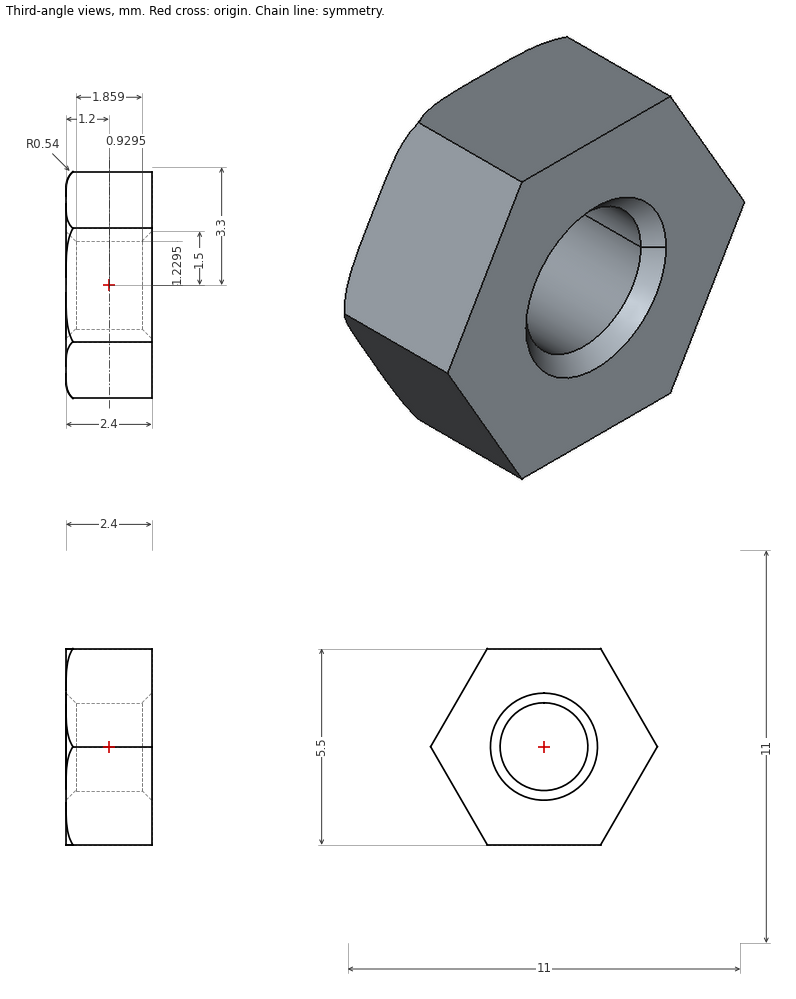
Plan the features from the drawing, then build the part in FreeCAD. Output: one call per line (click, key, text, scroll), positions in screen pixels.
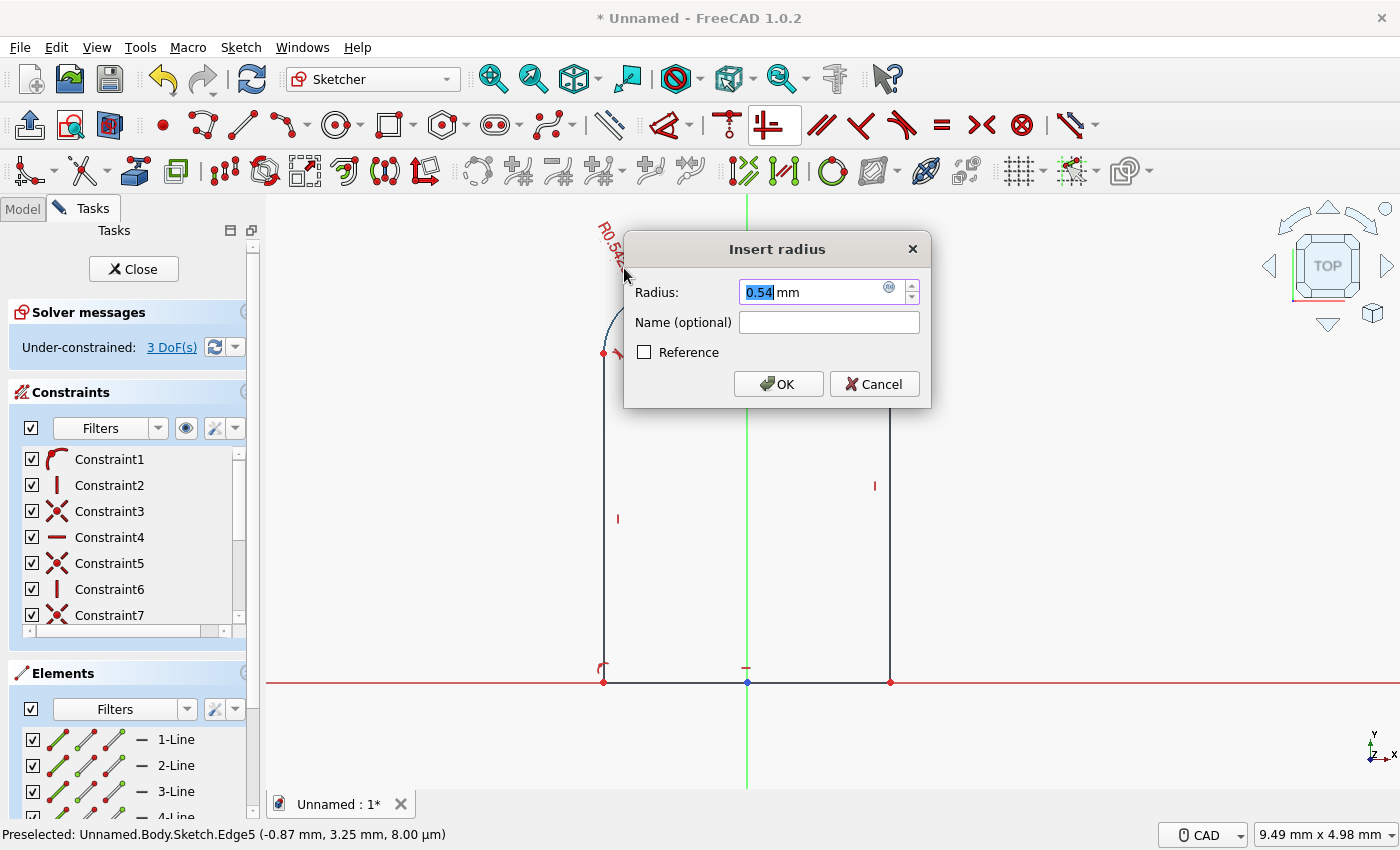
text(0.54)
key(Return)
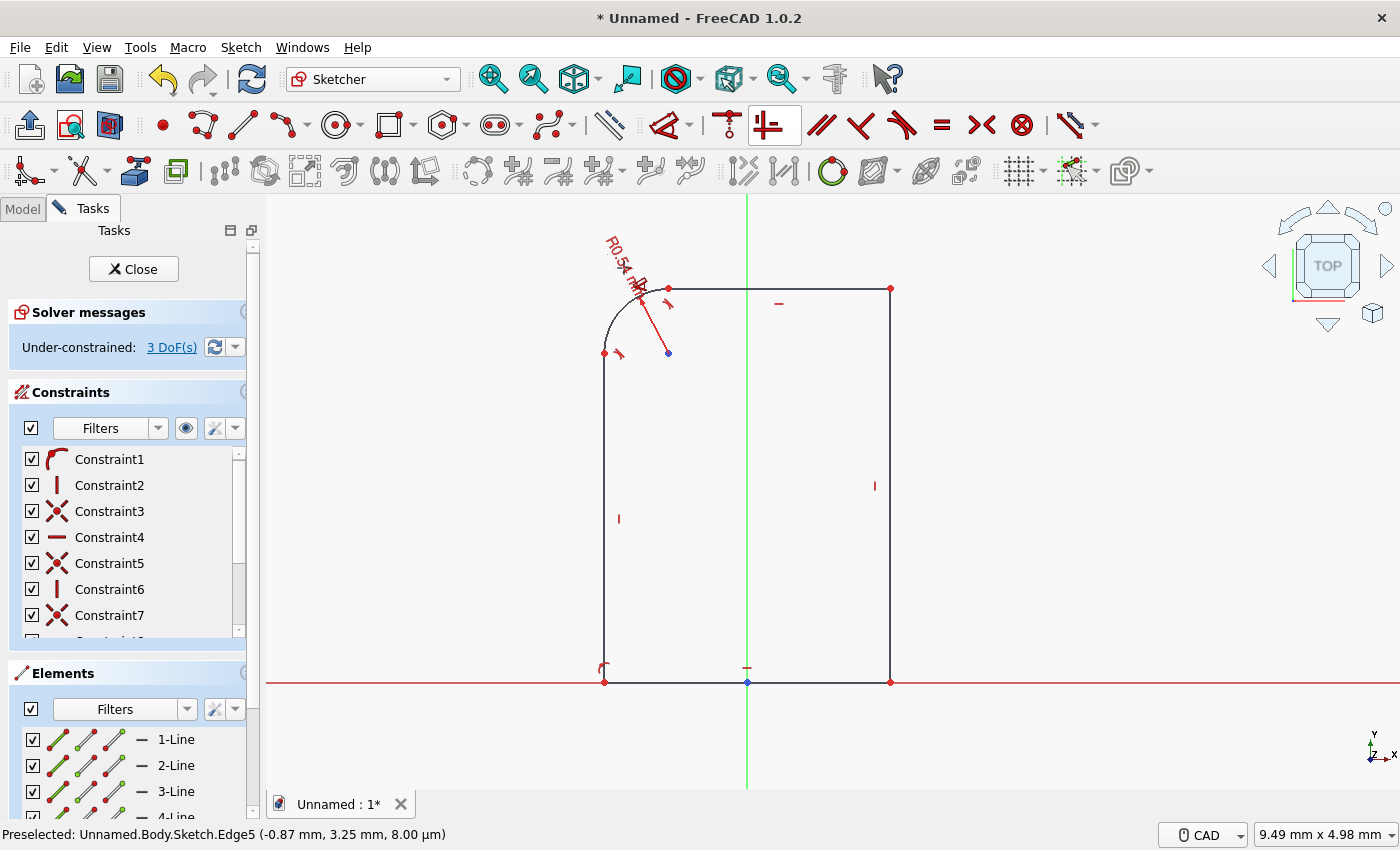
click(690, 683)
click(681, 717)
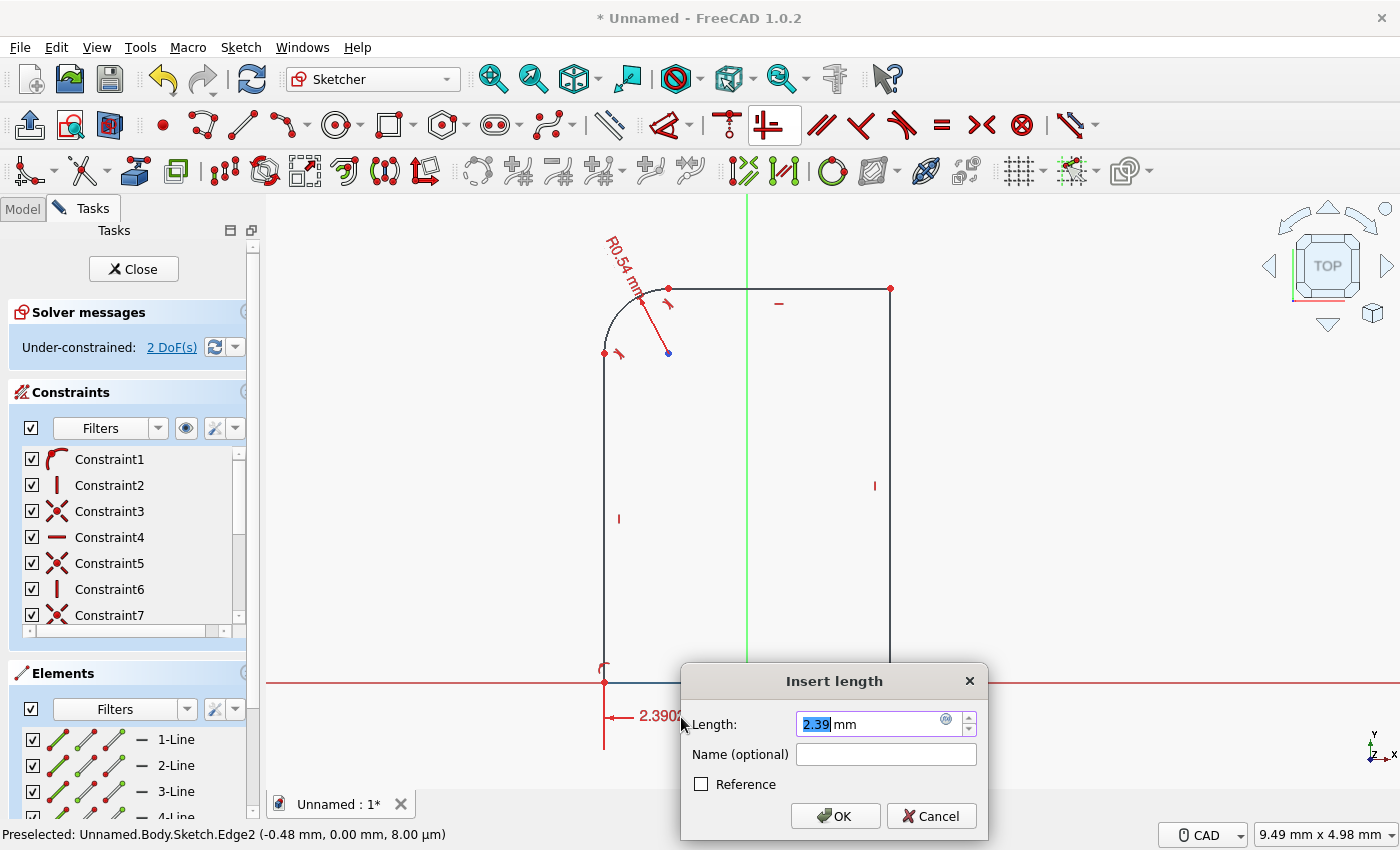
text(2.4)
key(Return)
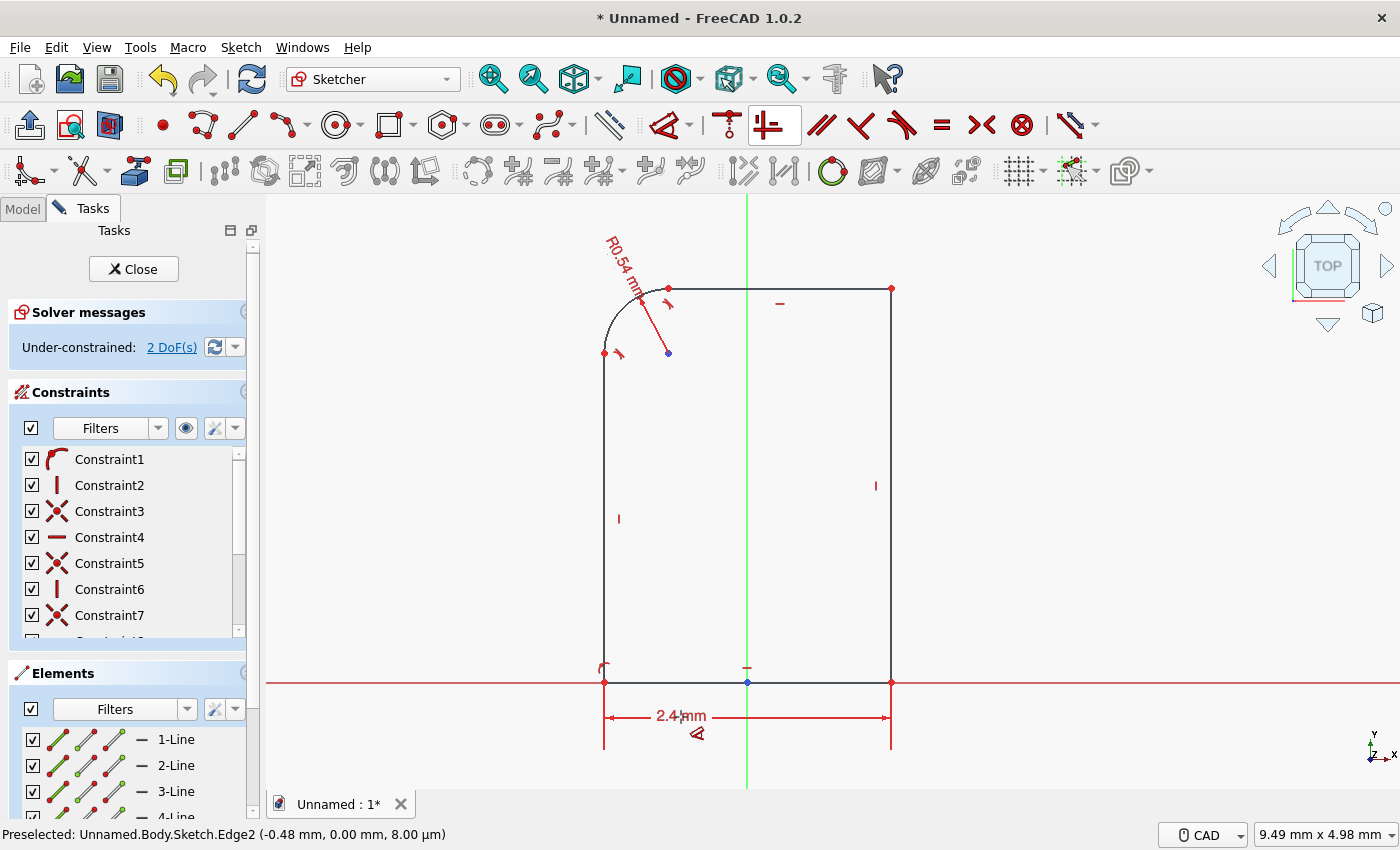
click(891, 565)
click(925, 486)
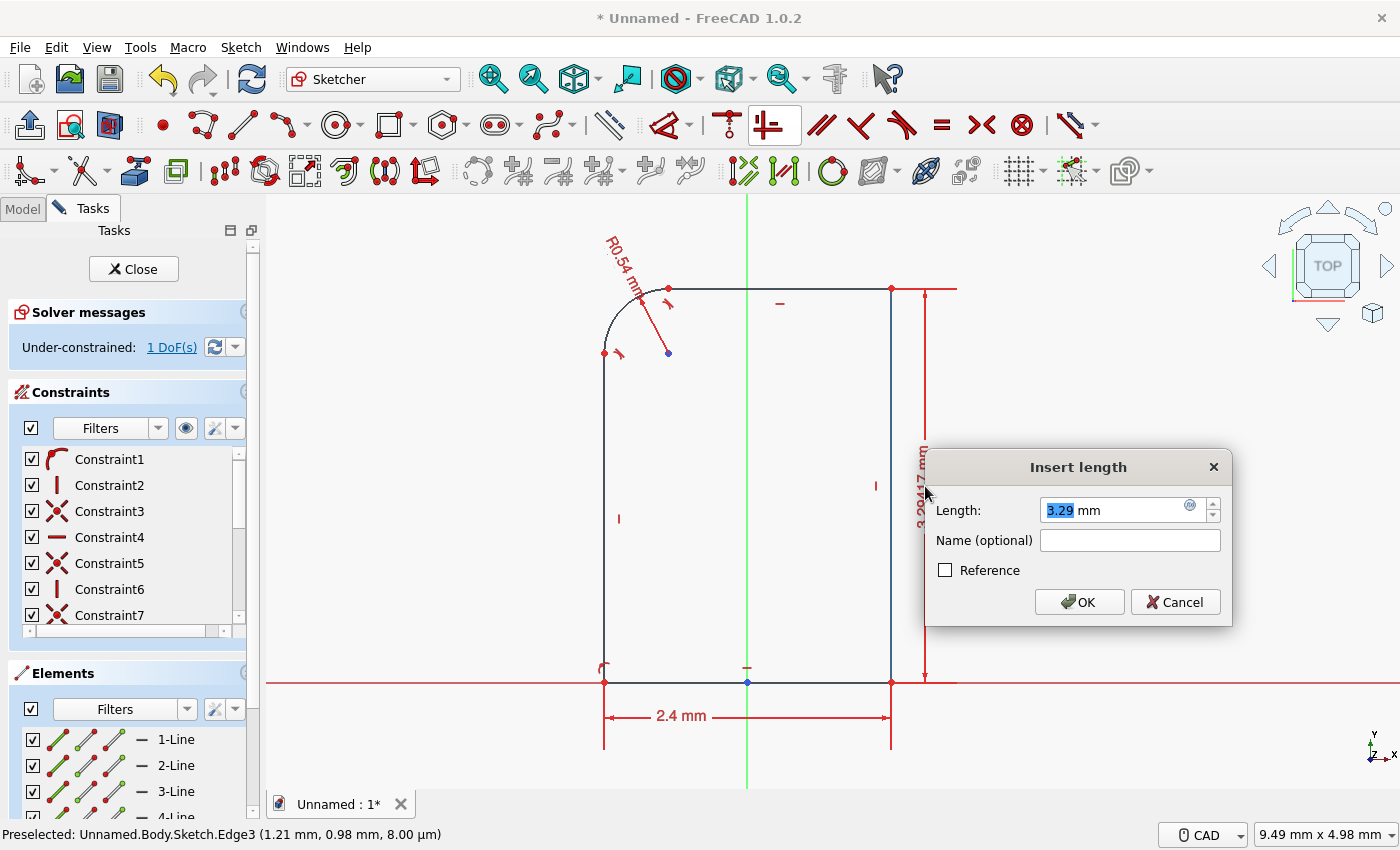
text(3.3)
key(Return)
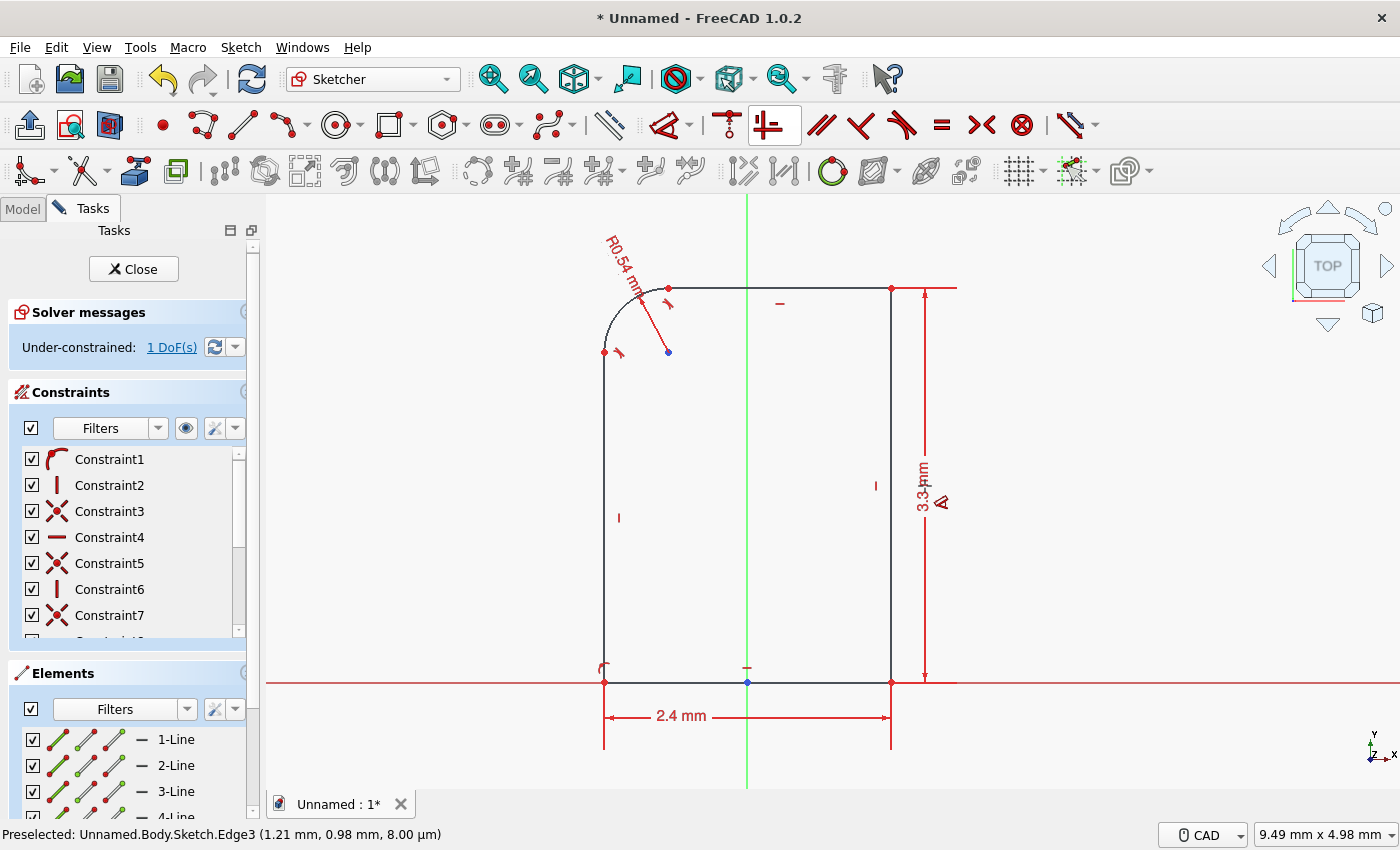
click(604, 353)
click(676, 319)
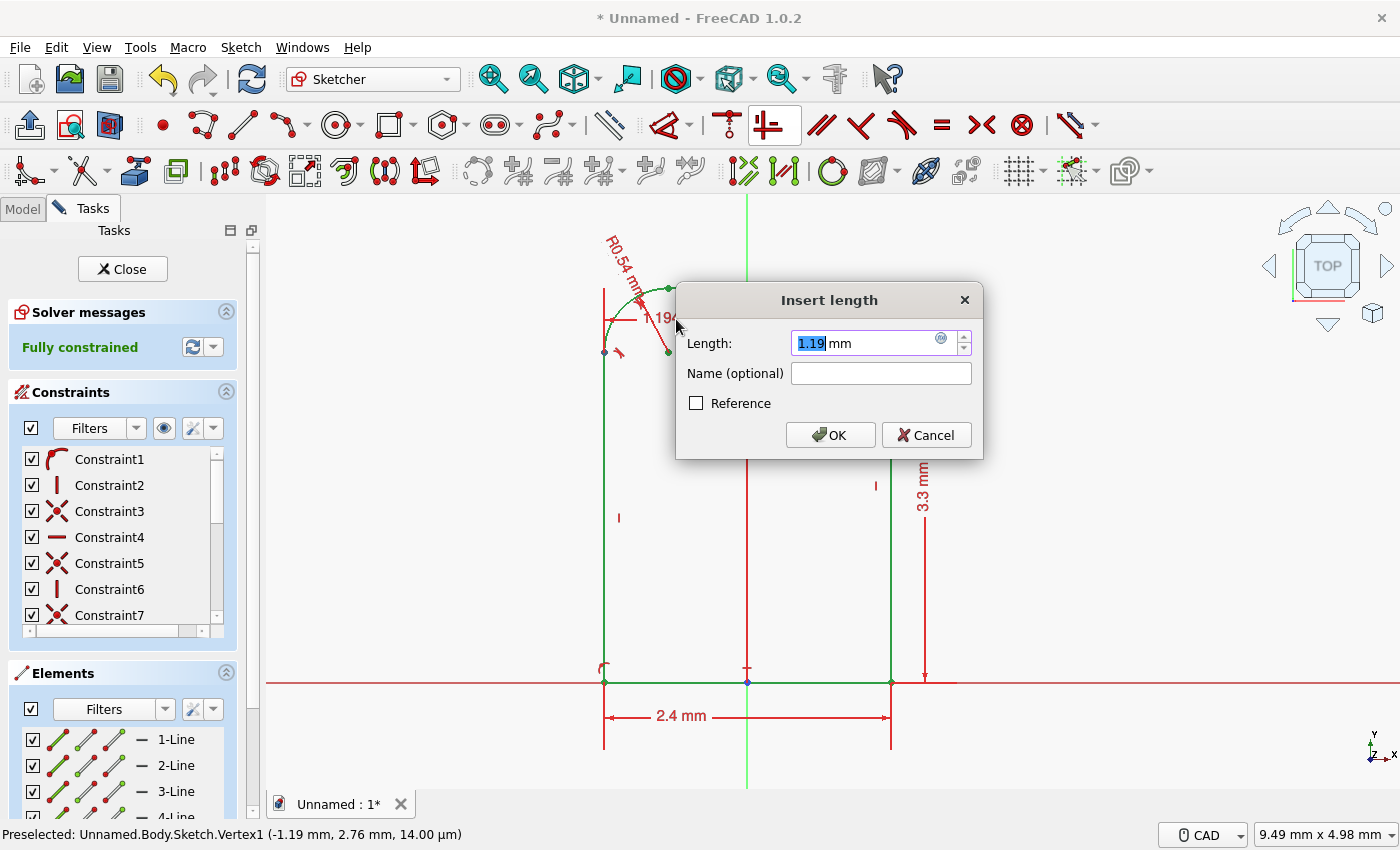
text(1.2)
key(Return)
key(Escape)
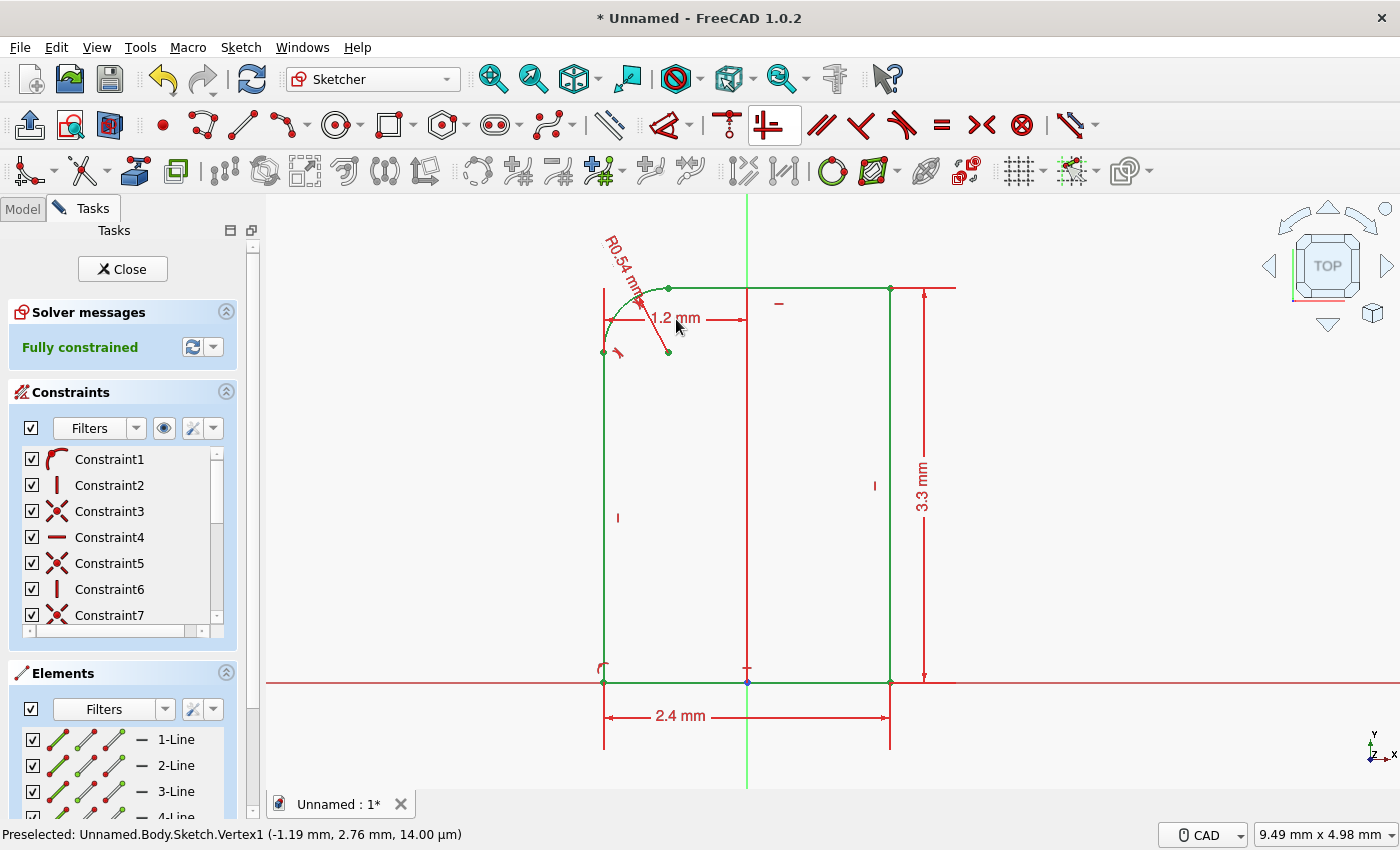
click(123, 269)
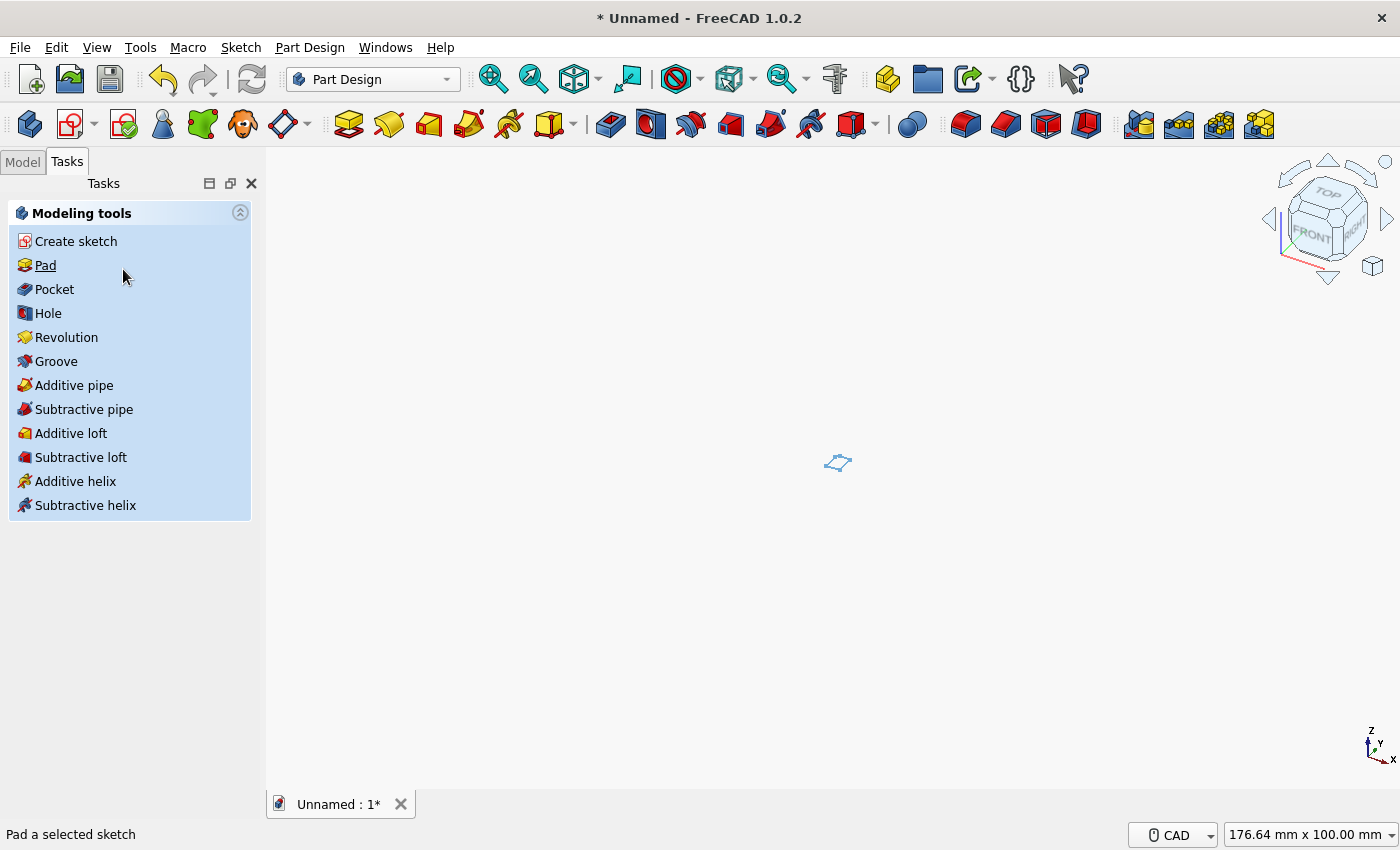
click(390, 124)